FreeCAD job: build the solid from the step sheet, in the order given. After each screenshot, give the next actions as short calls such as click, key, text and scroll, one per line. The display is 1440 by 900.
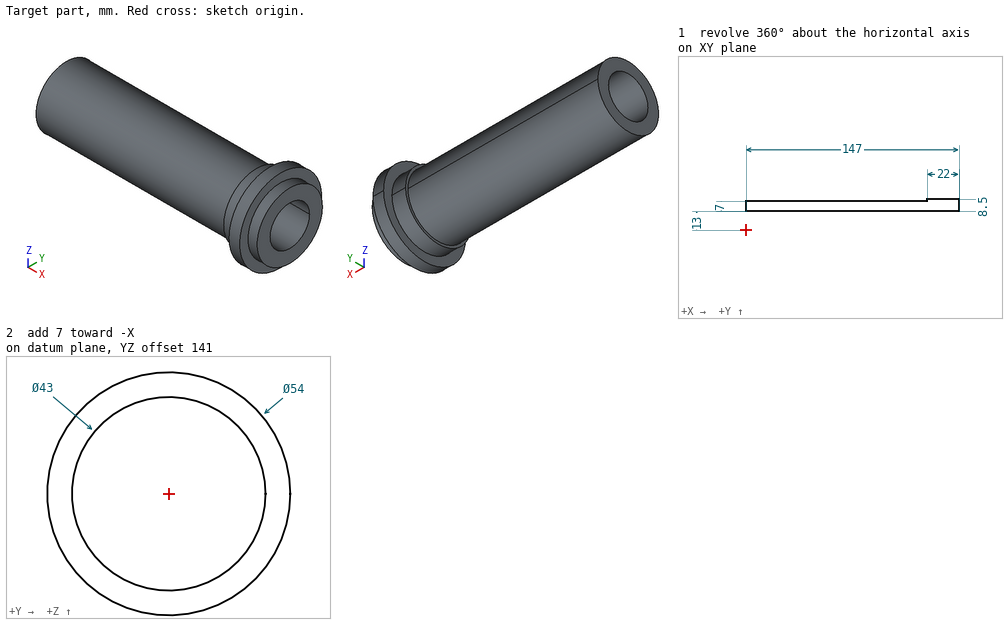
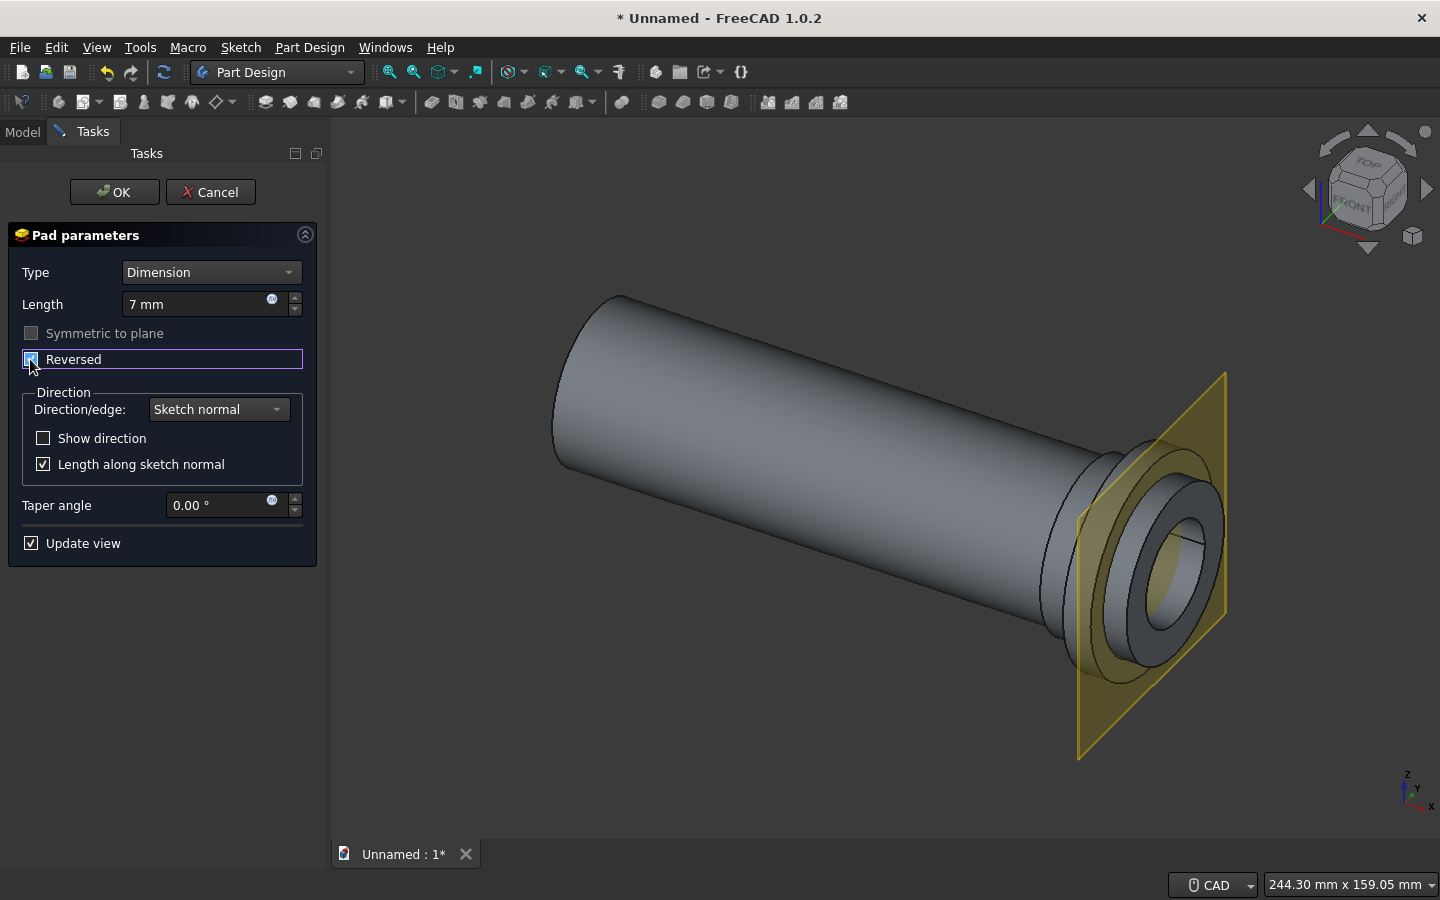
click(115, 192)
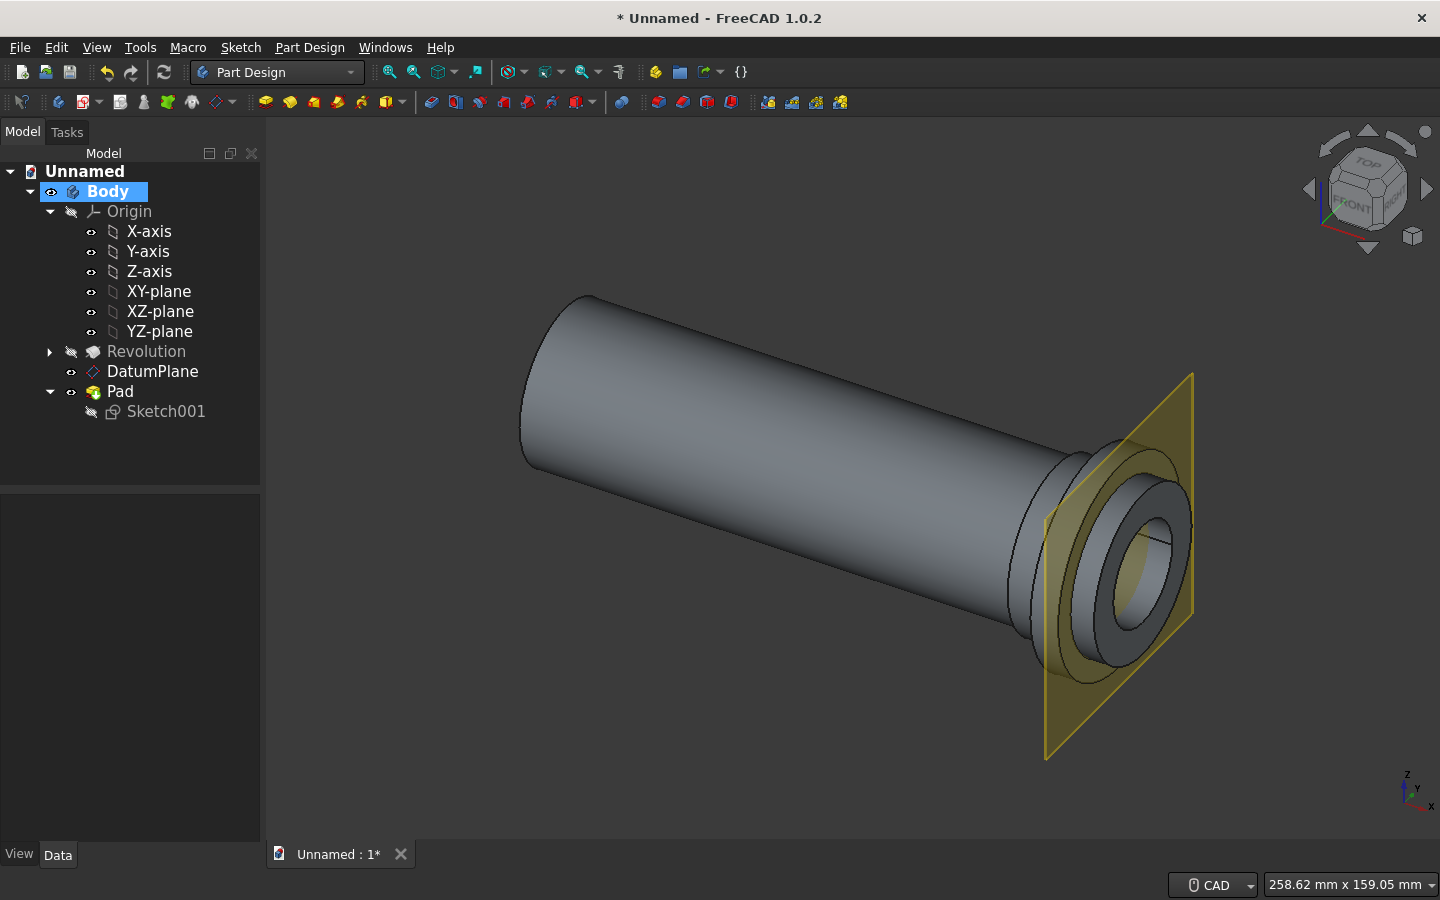
click(116, 372)
key(space)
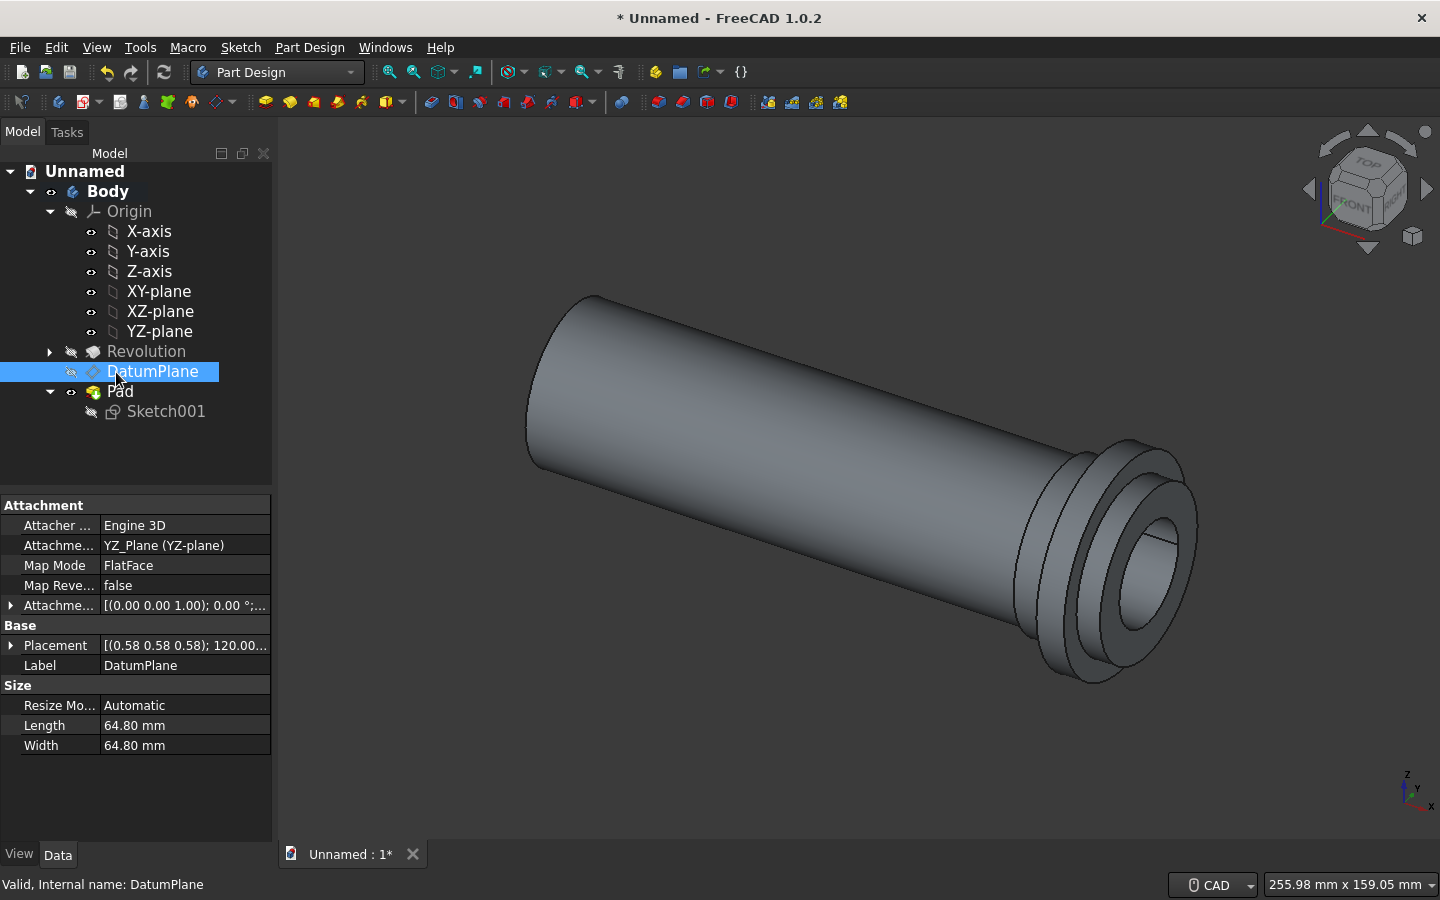
key(0)